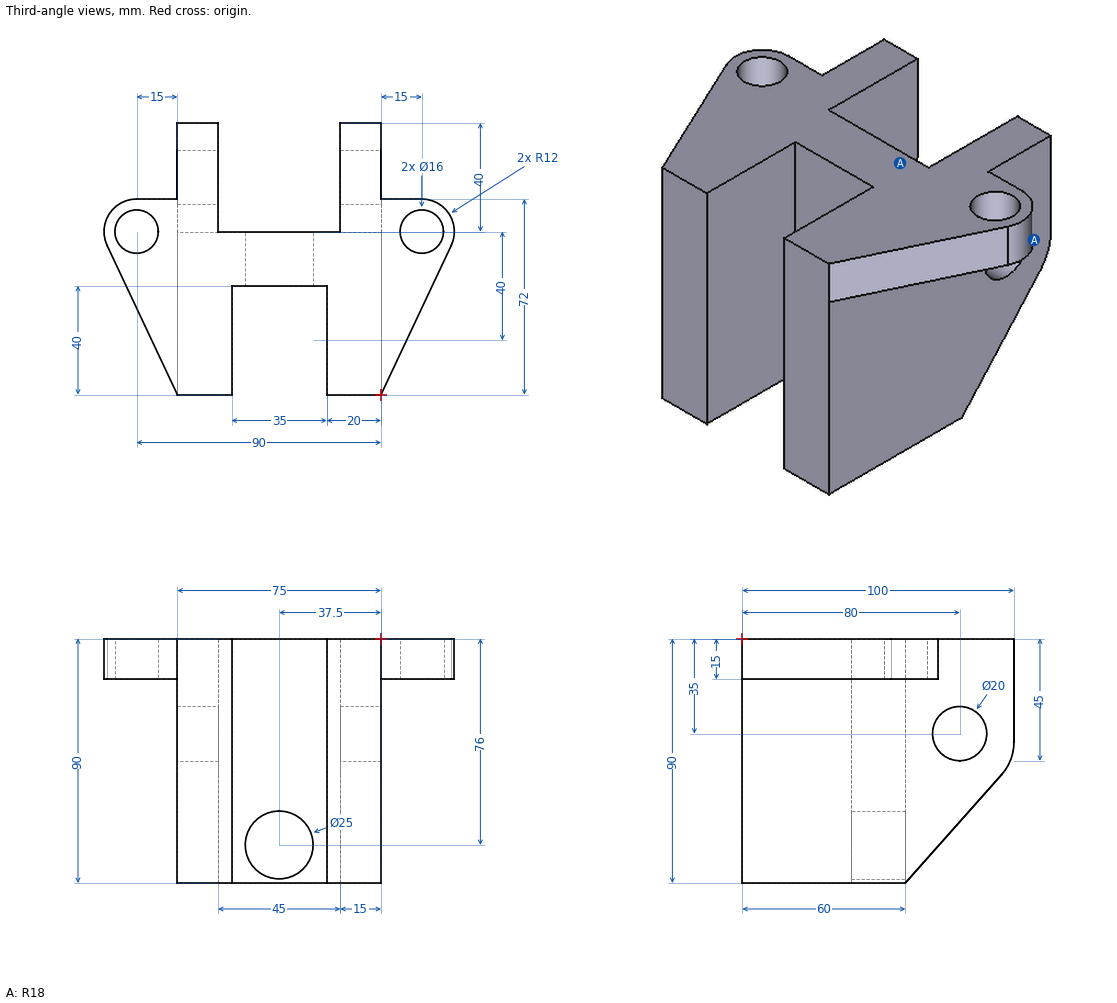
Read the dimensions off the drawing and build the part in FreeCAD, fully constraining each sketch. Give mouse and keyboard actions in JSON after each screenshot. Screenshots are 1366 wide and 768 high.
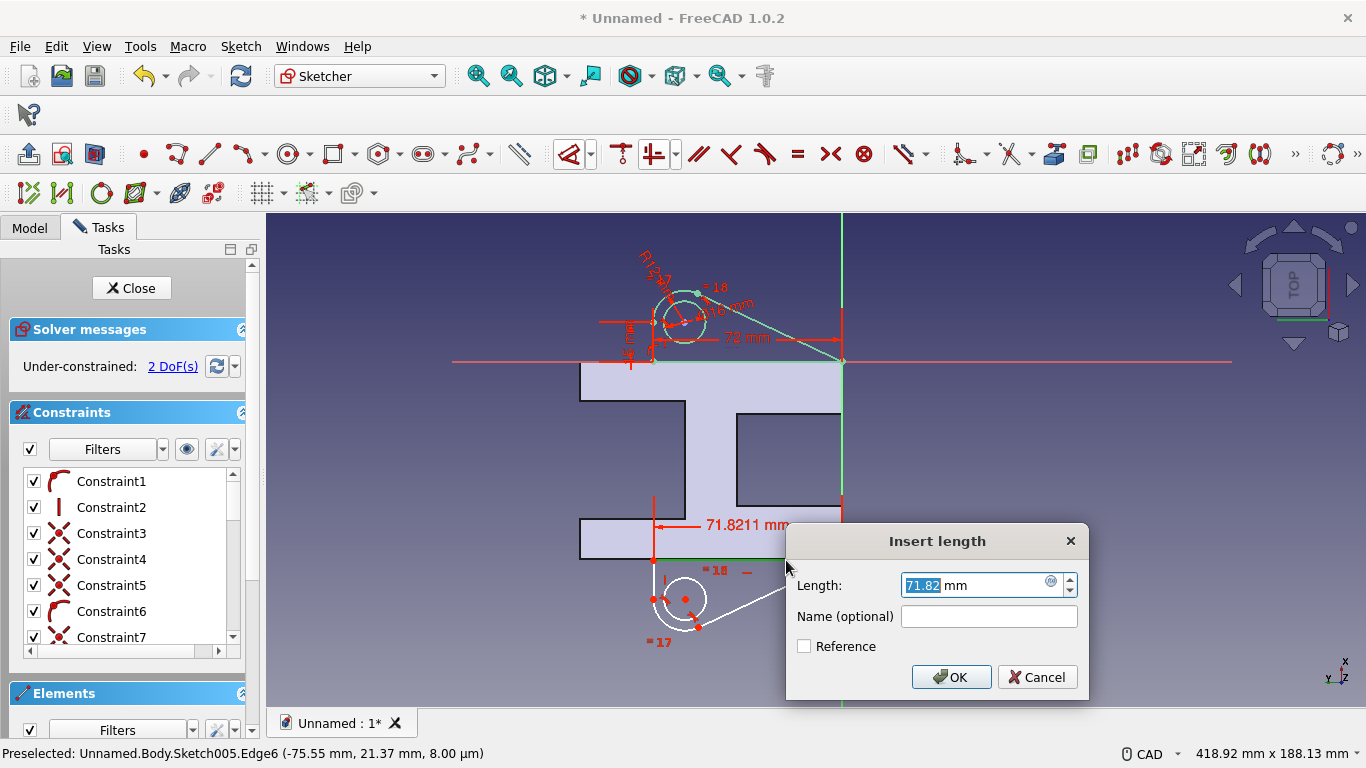
{"action": "type", "text": "72"}
{"action": "key", "text": "Return"}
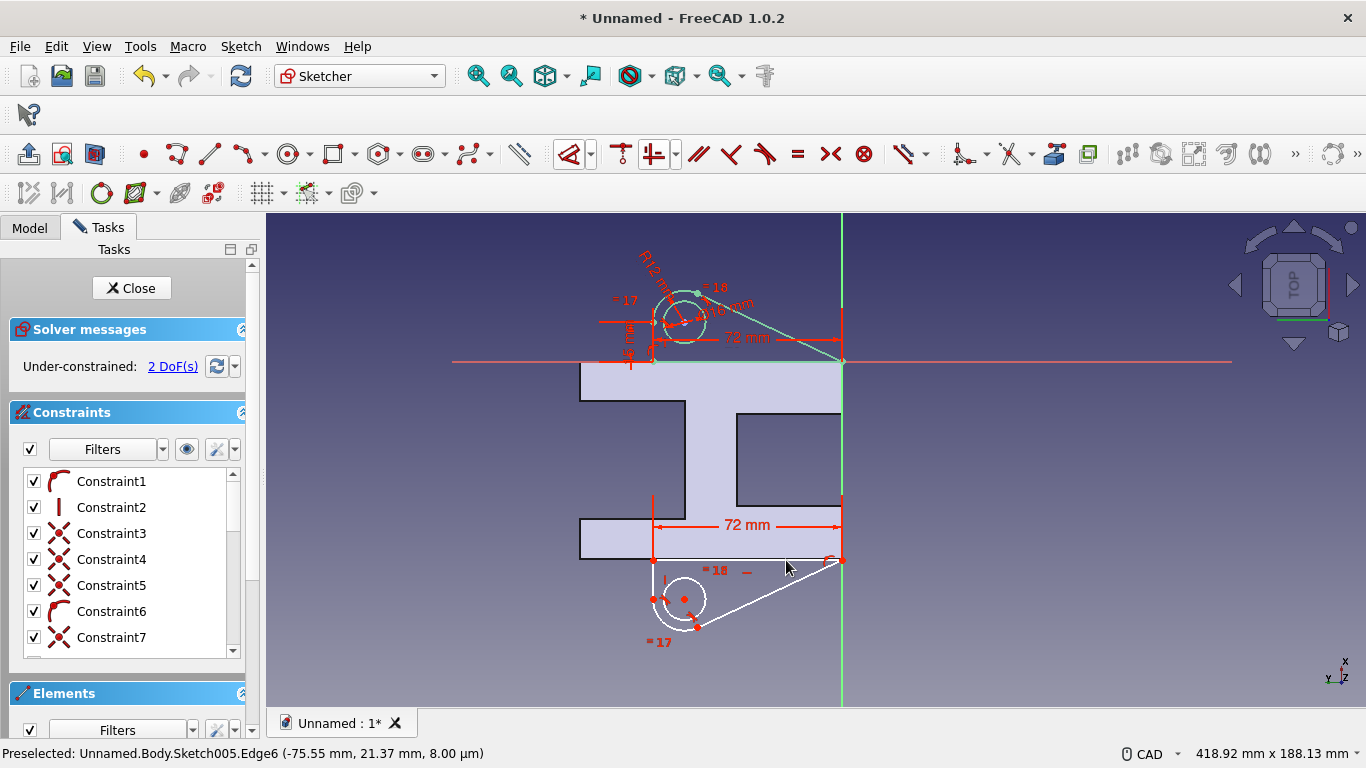
{"action": "left_click", "coordinate": [653, 572]}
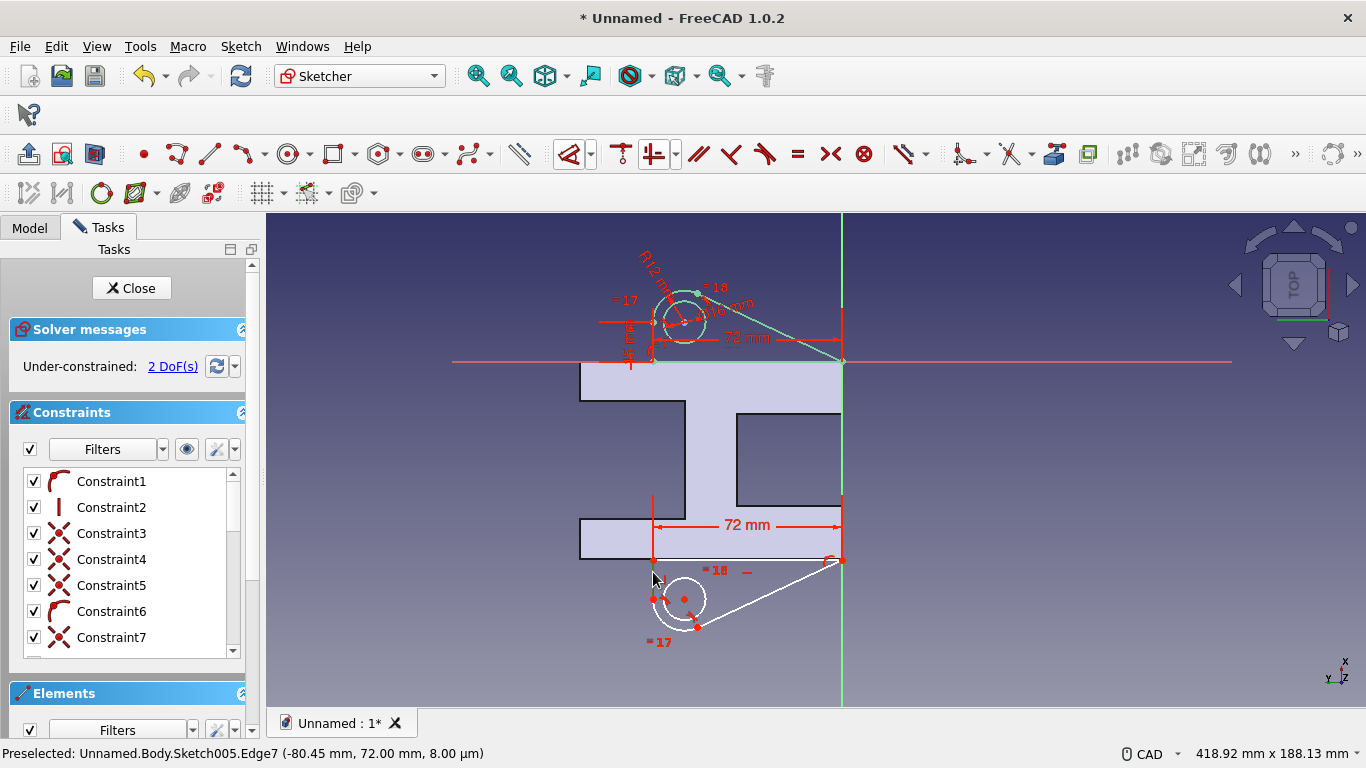
{"action": "key", "text": "i"}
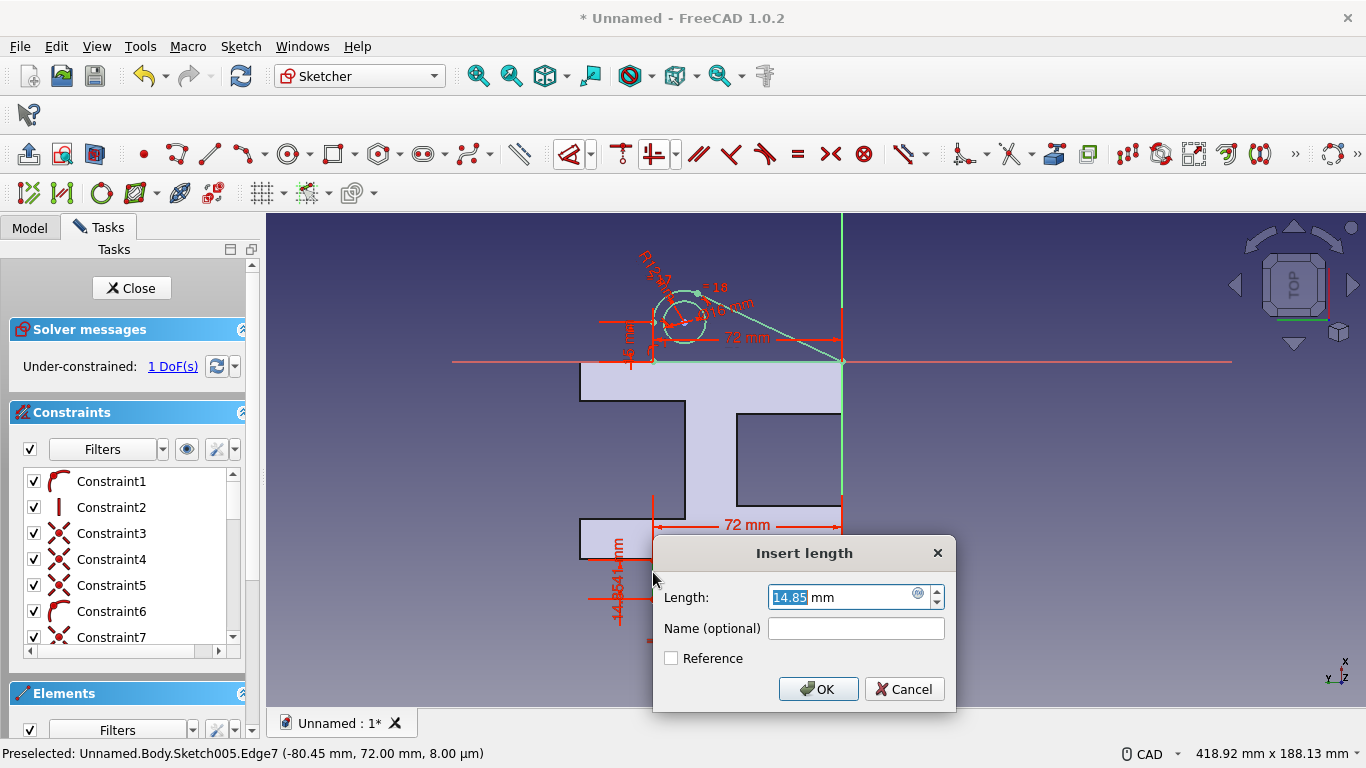
{"action": "type", "text": "15"}
{"action": "key", "text": "Return"}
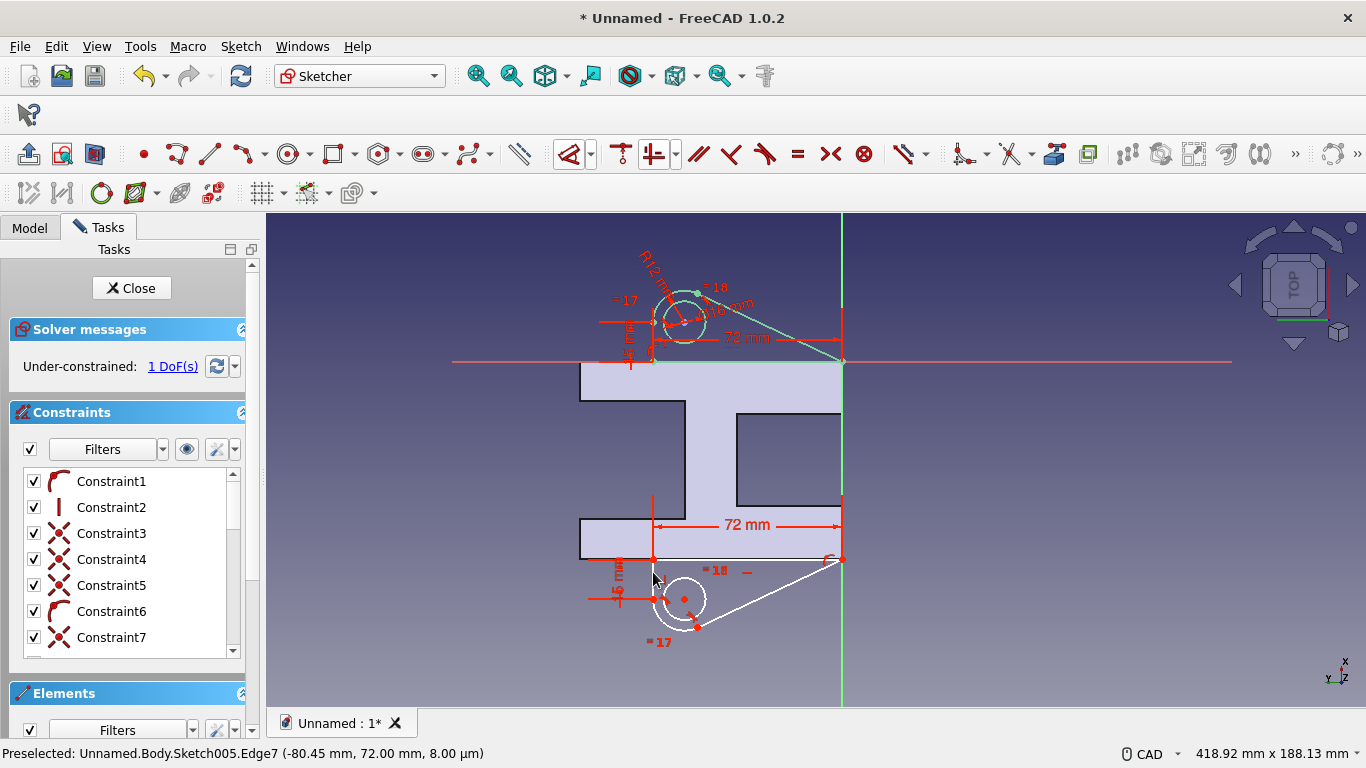
{"action": "left_click", "coordinate": [685, 599]}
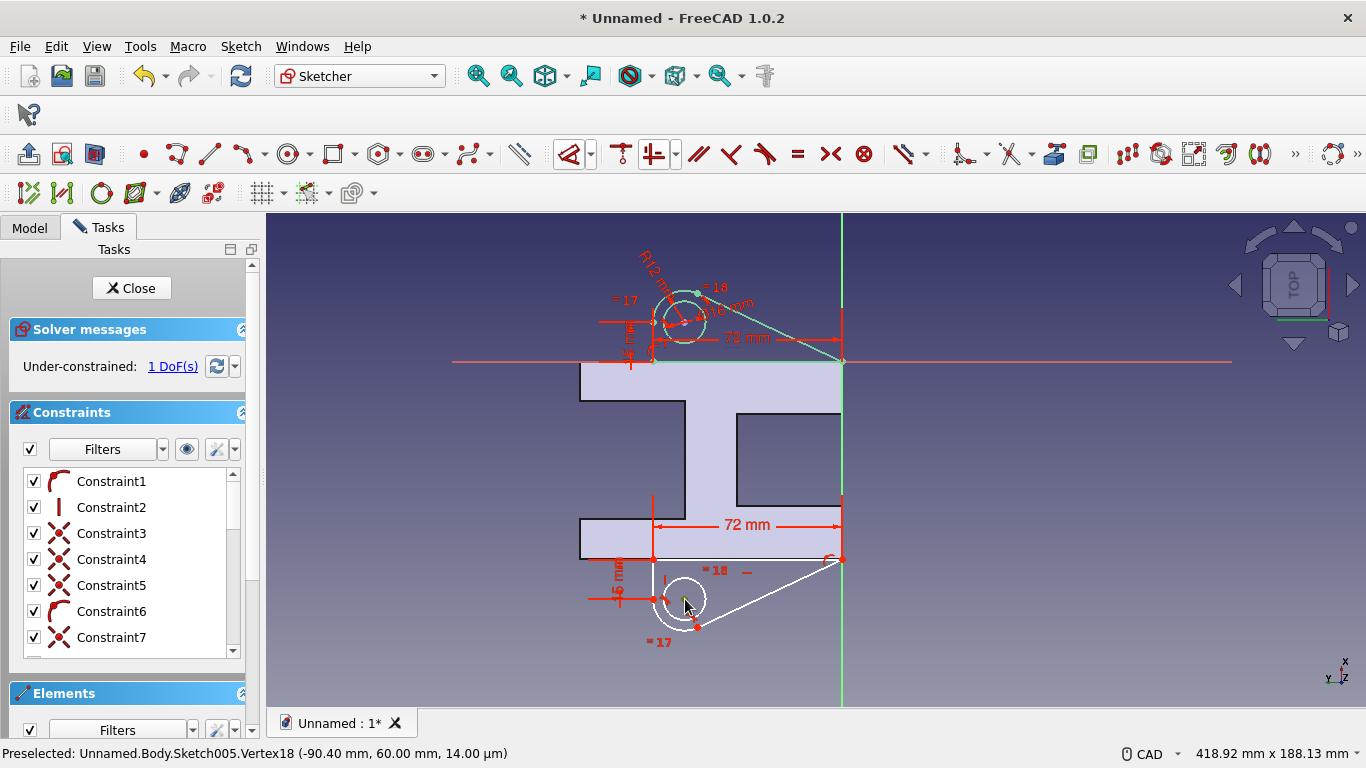
{"action": "key", "text": "i"}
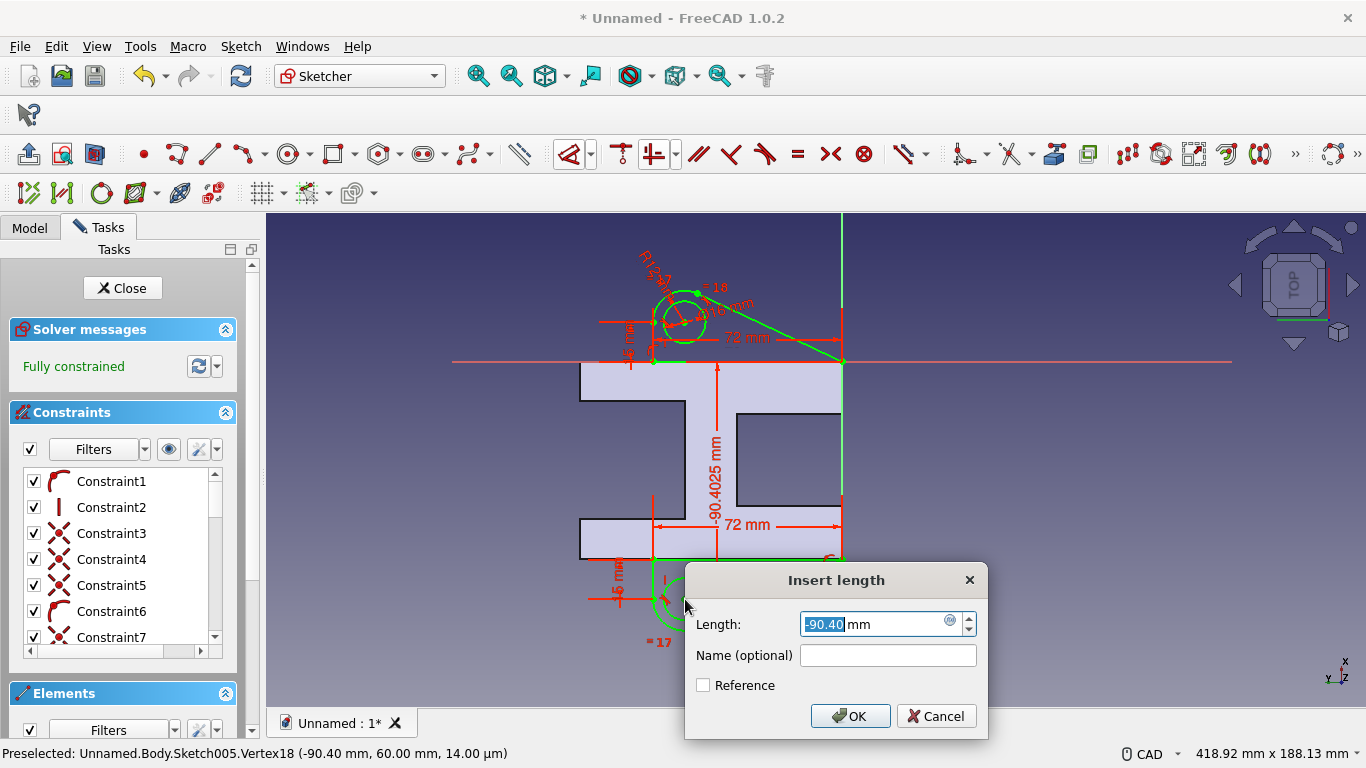
{"action": "type", "text": "-90"}
{"action": "key", "text": "Return"}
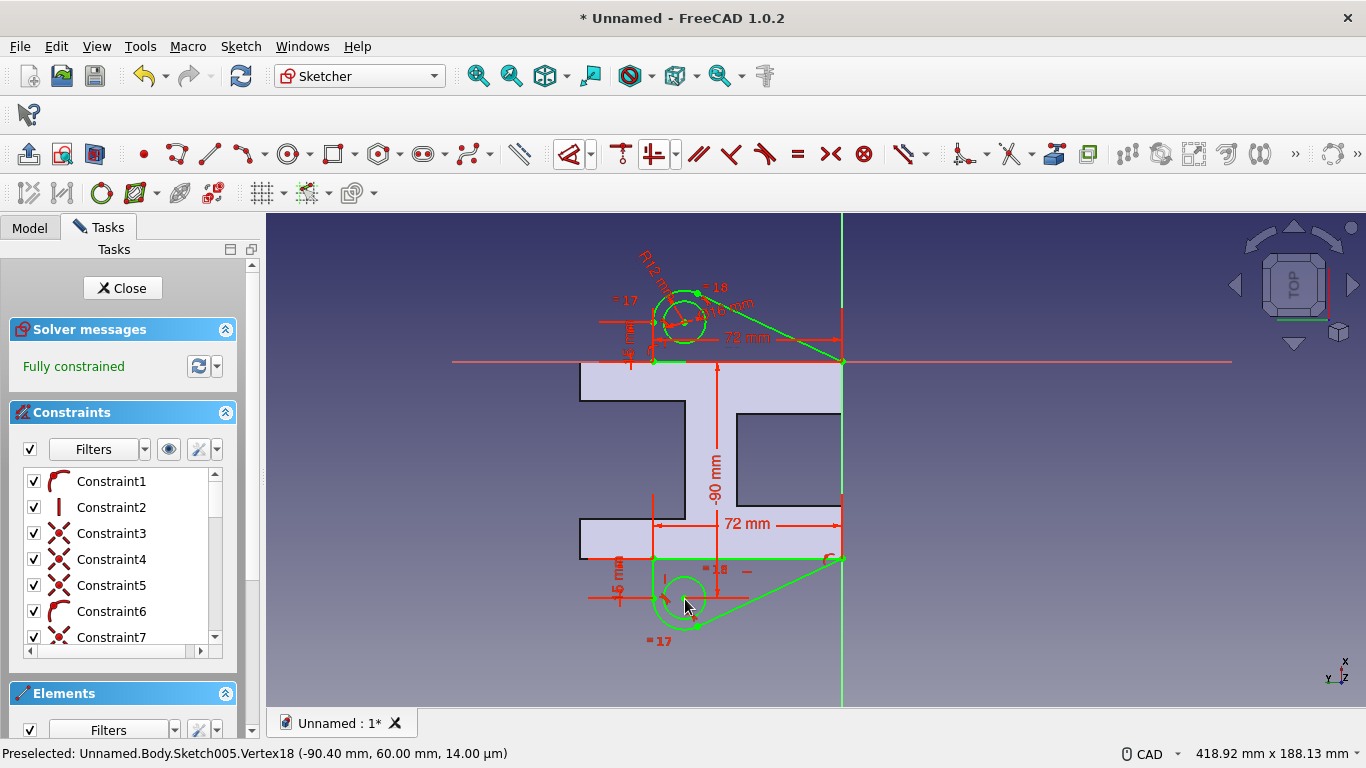
{"action": "left_click", "coordinate": [123, 288]}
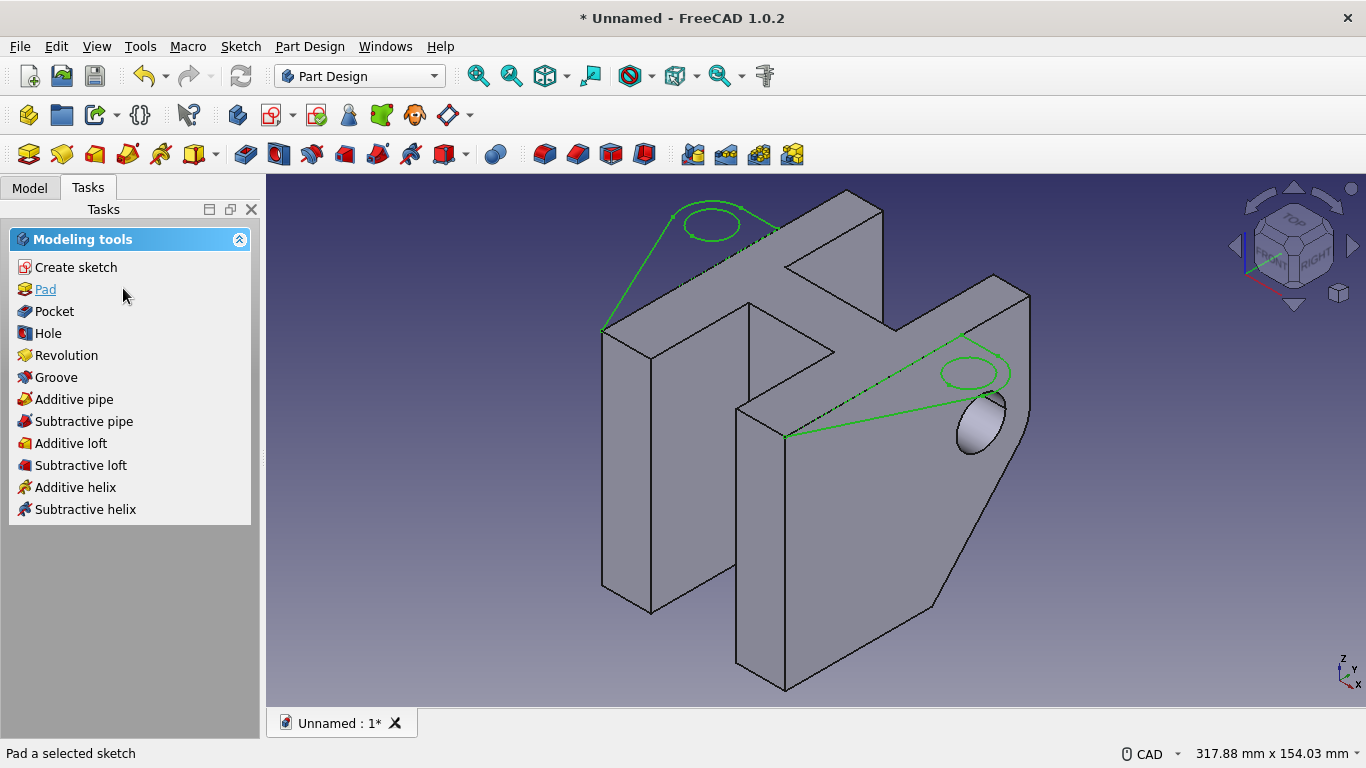
{"action": "left_click", "coordinate": [29, 154]}